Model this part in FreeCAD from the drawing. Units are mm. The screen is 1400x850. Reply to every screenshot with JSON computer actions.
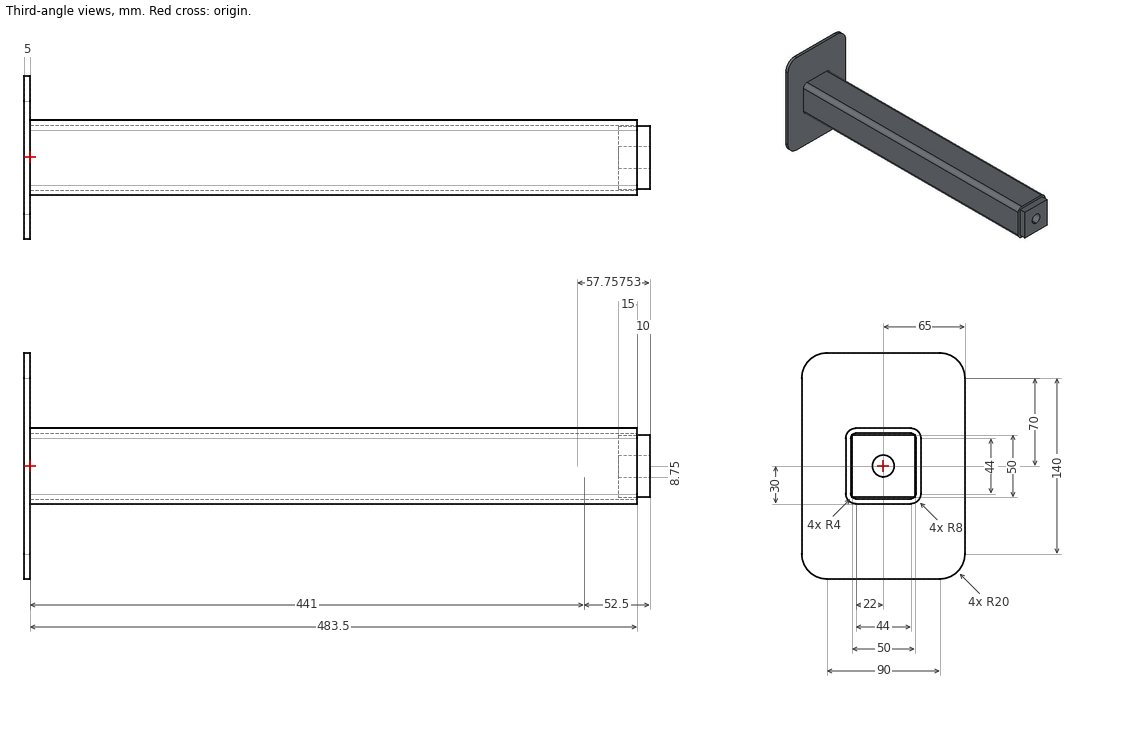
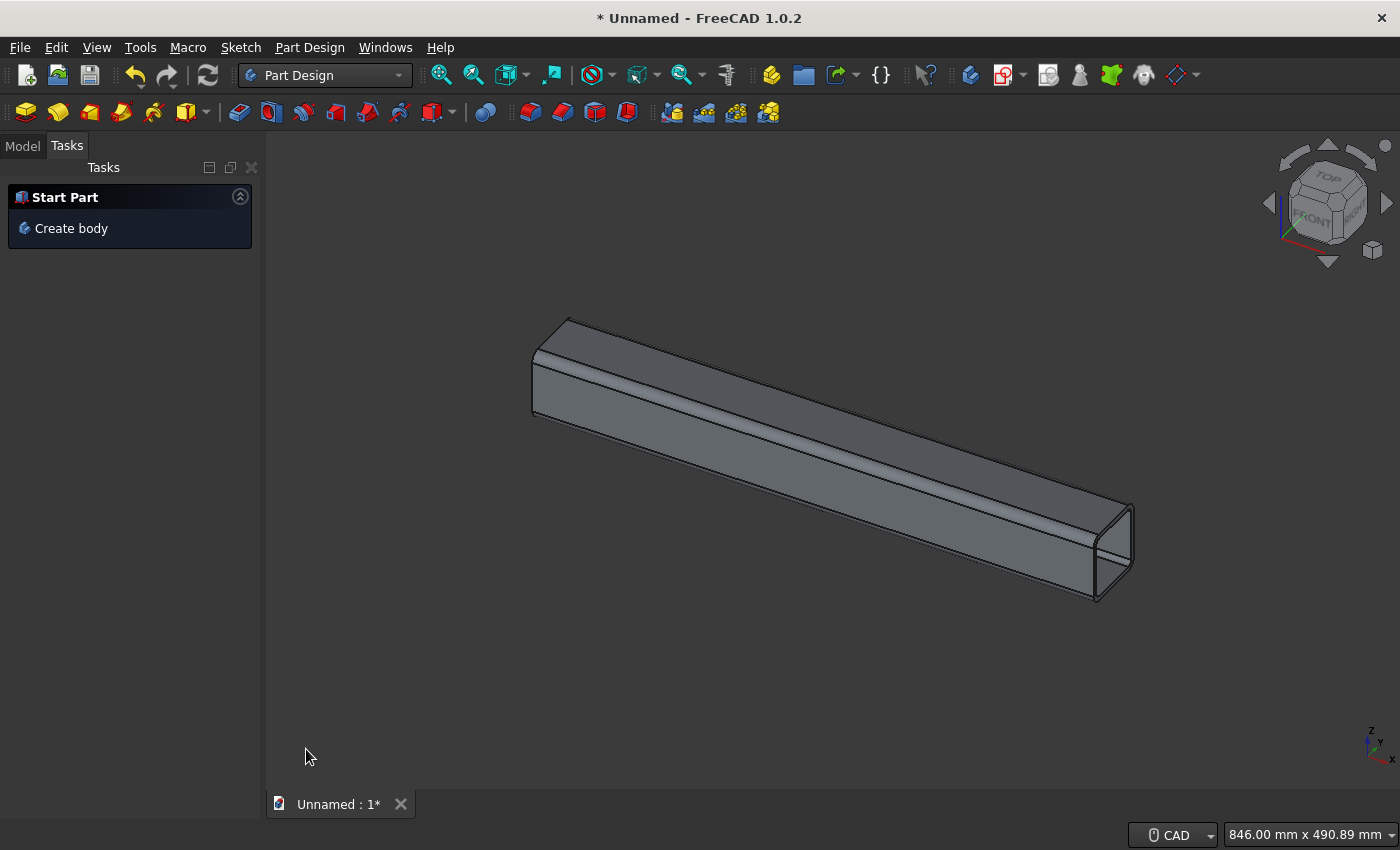
{"action": "left_click", "coordinate": [1004, 76]}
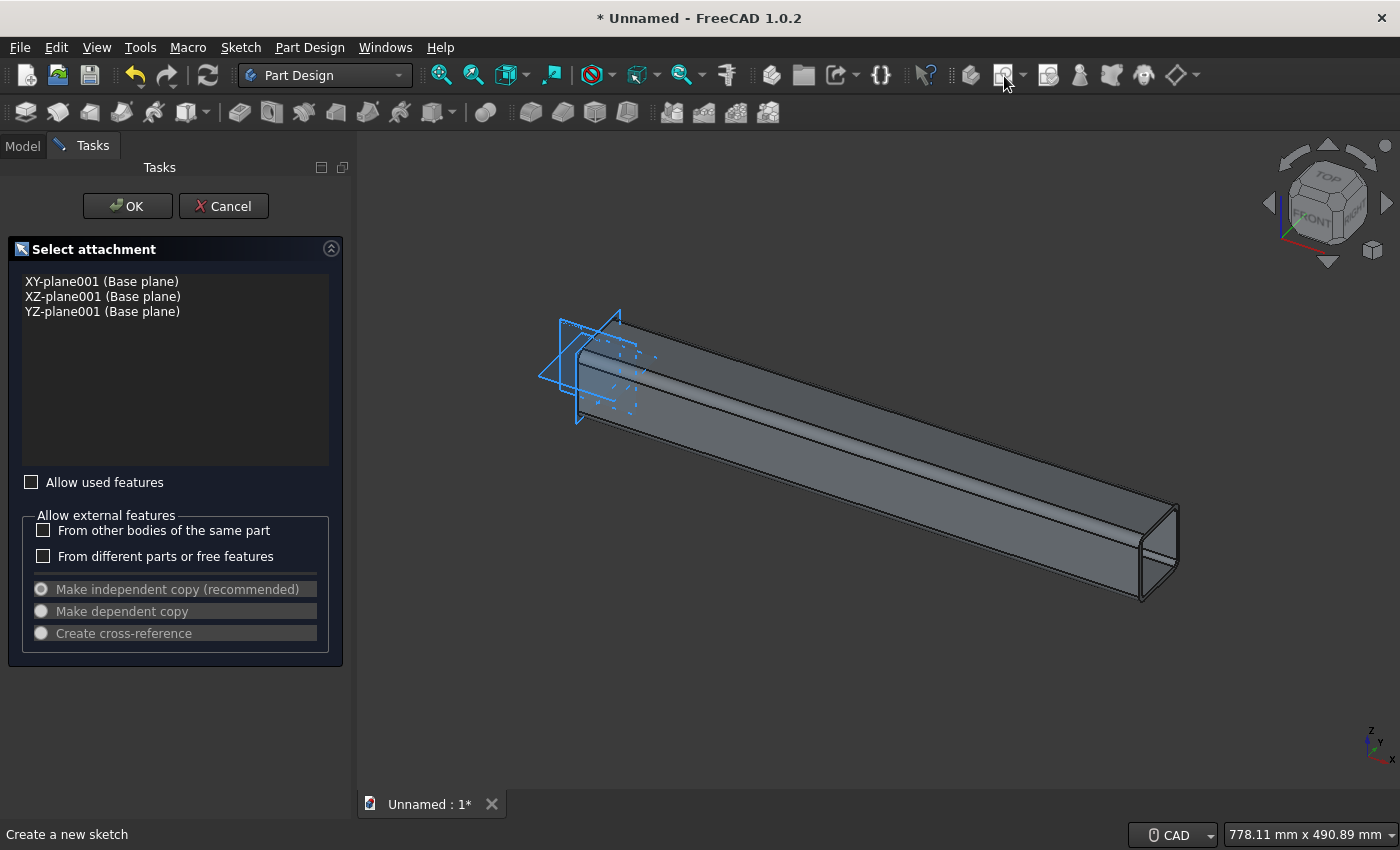
{"action": "left_click", "coordinate": [82, 312]}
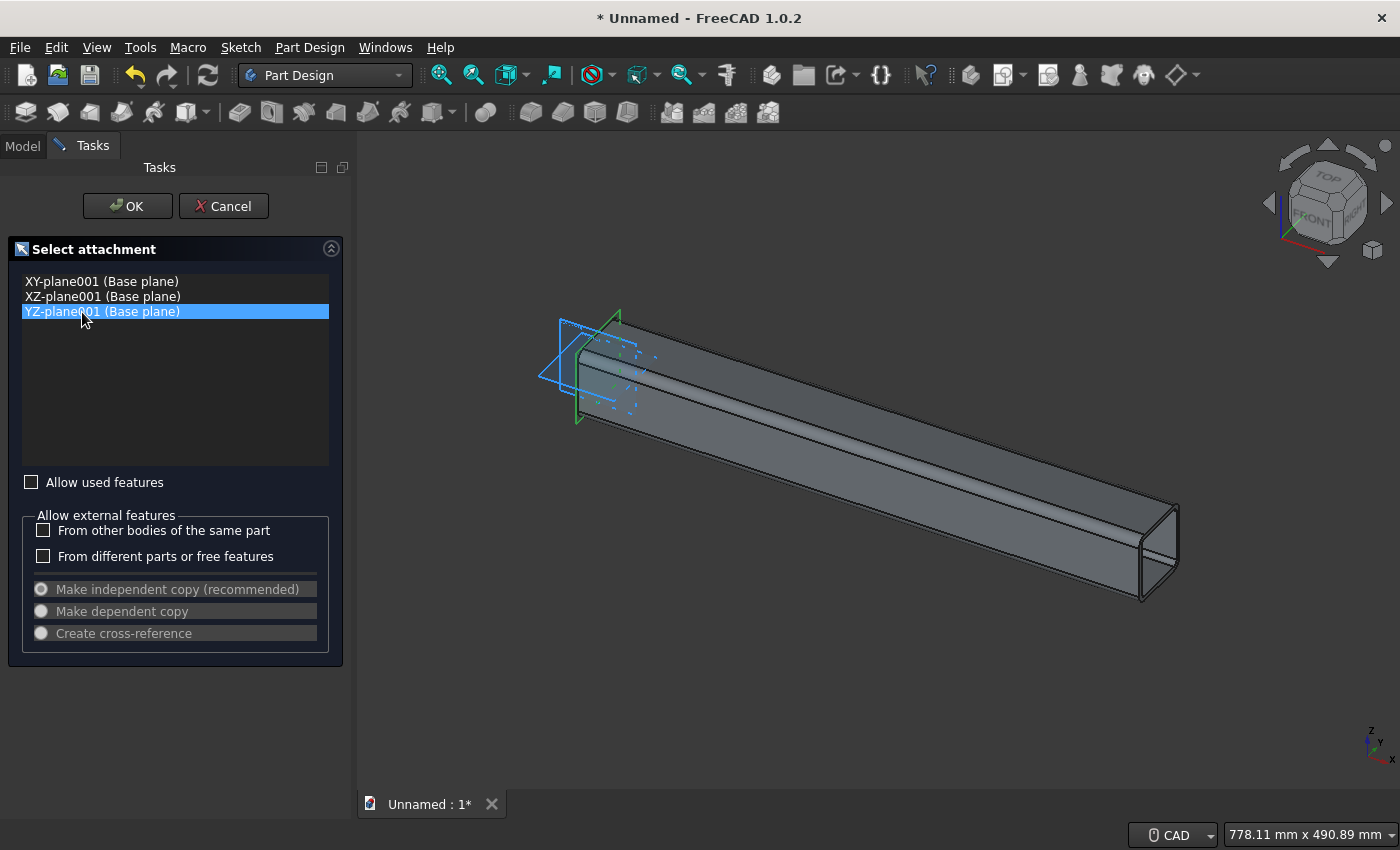
{"action": "left_click", "coordinate": [128, 206]}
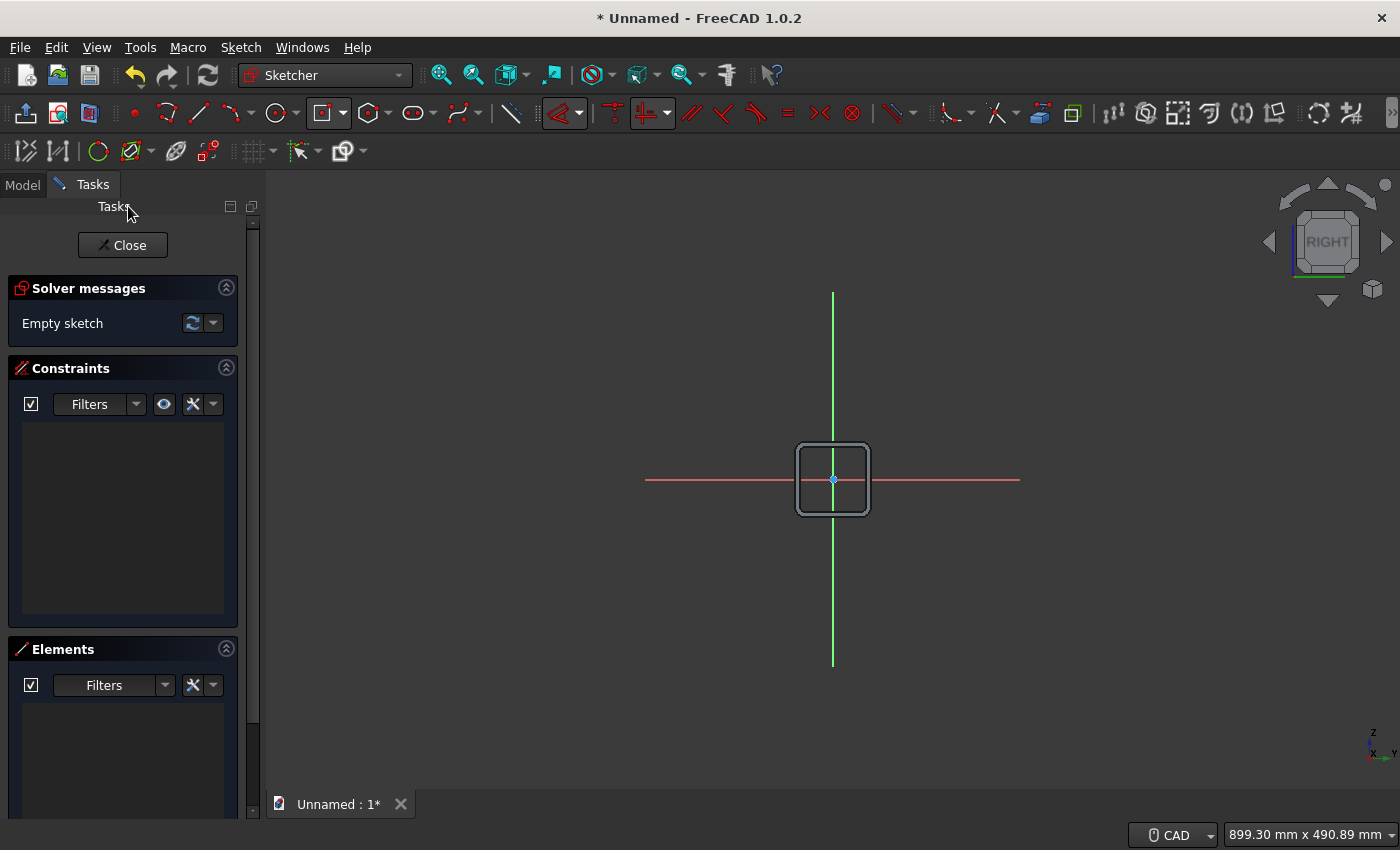
{"action": "scroll", "coordinate": [916, 480], "scroll_direction": "up", "scroll_amount": 3}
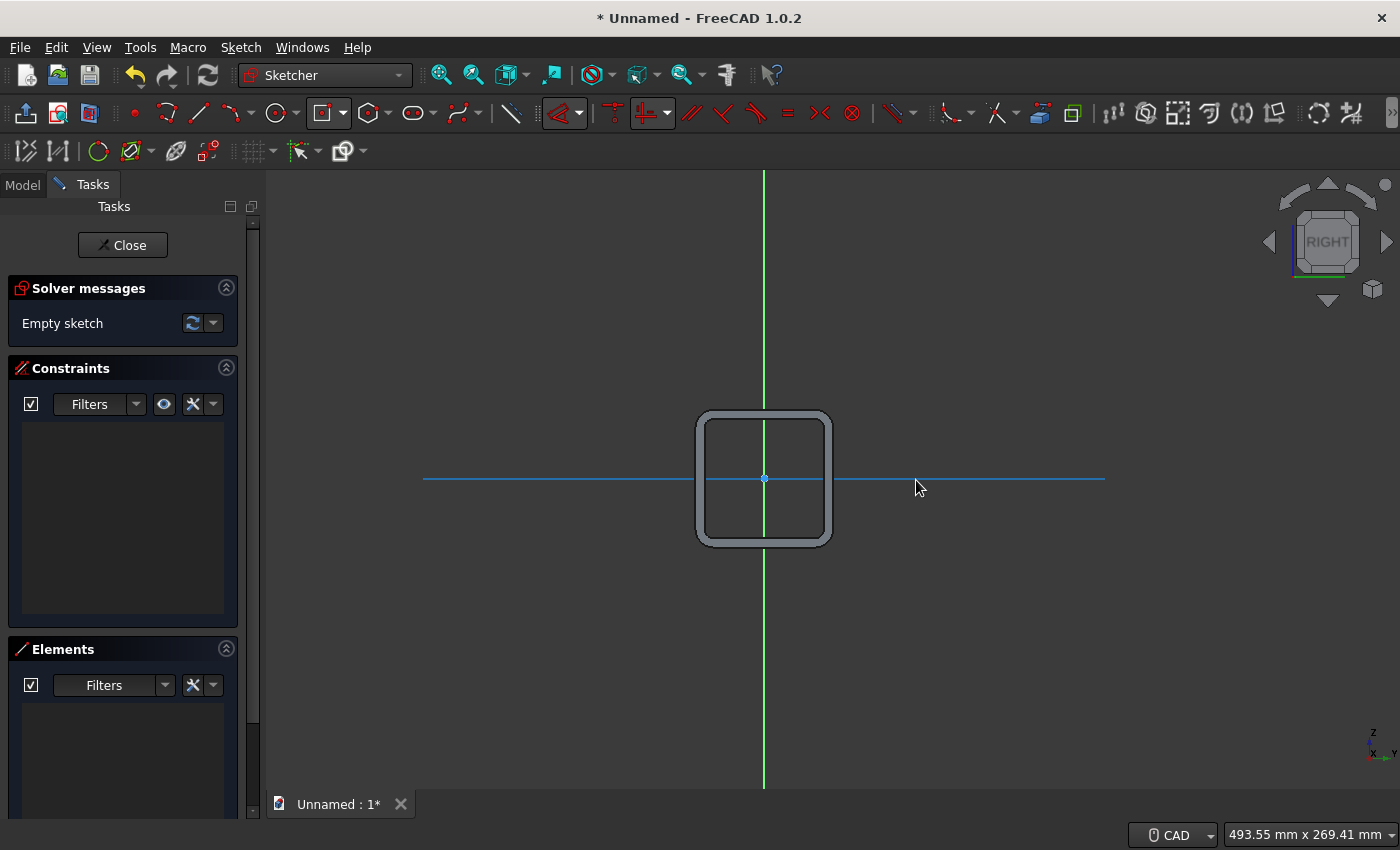
{"action": "left_click", "coordinate": [200, 114]}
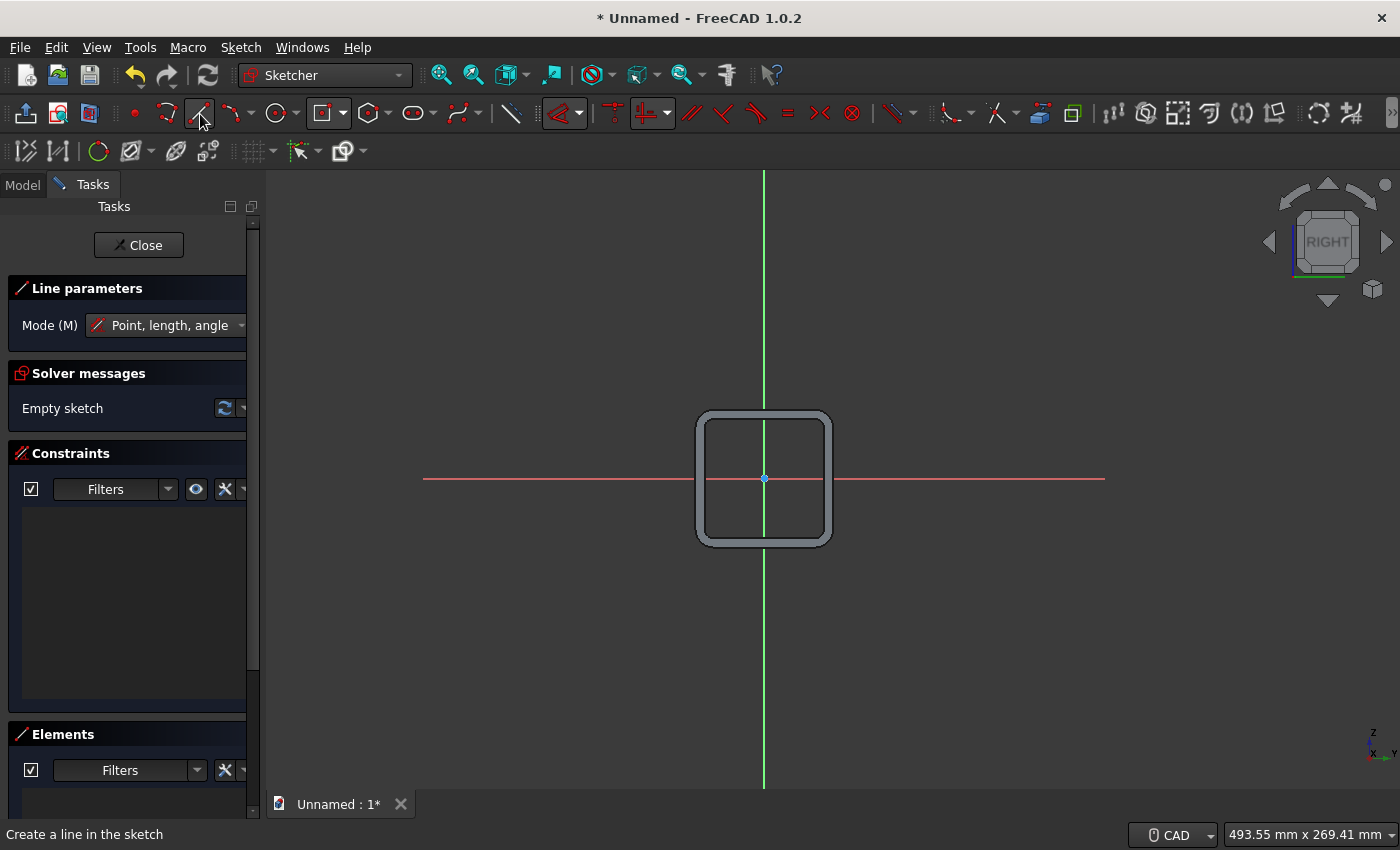
{"action": "left_click", "coordinate": [914, 318]}
{"action": "left_click", "coordinate": [914, 640]}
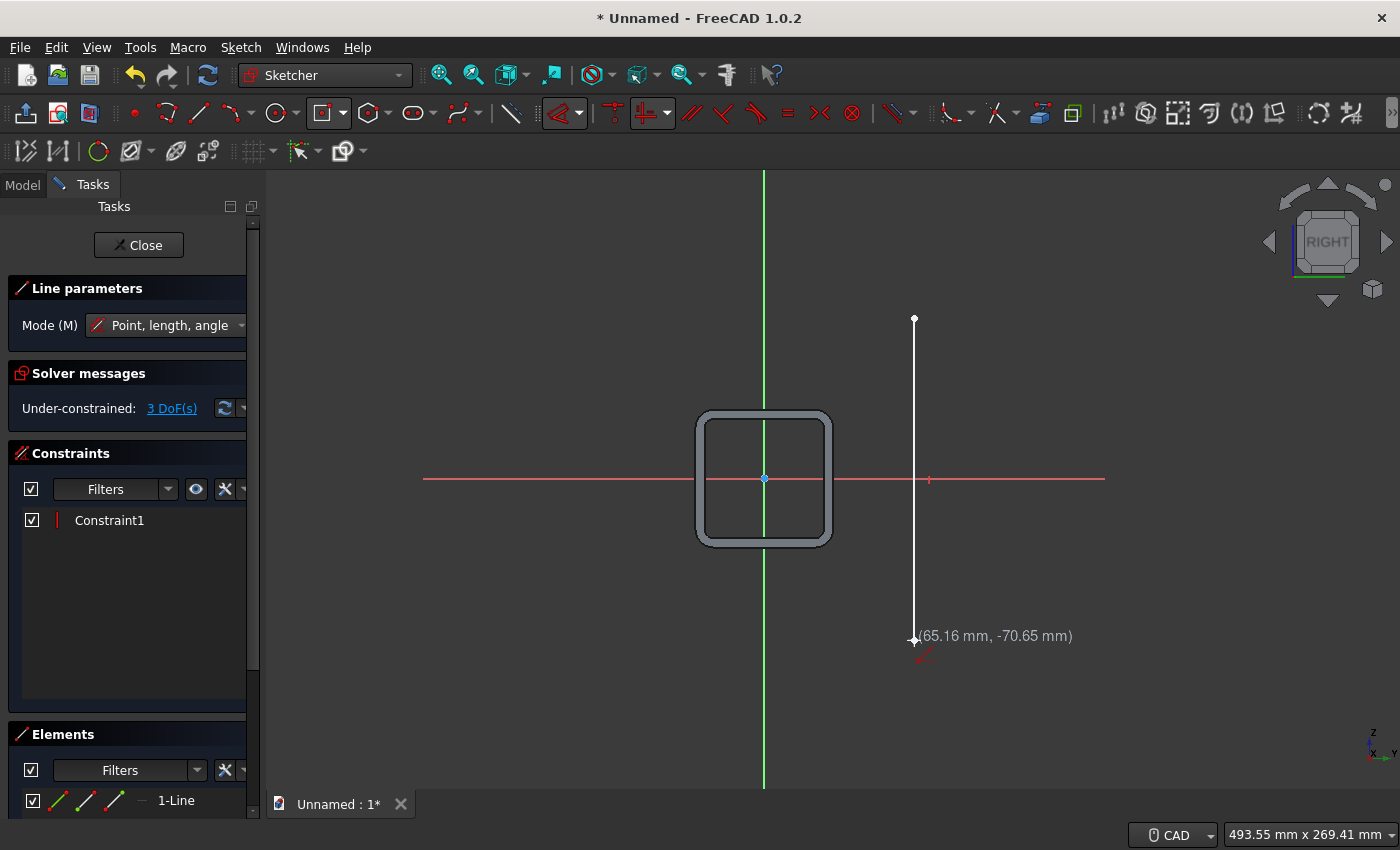
{"action": "left_click", "coordinate": [868, 685]}
{"action": "left_click", "coordinate": [661, 685]}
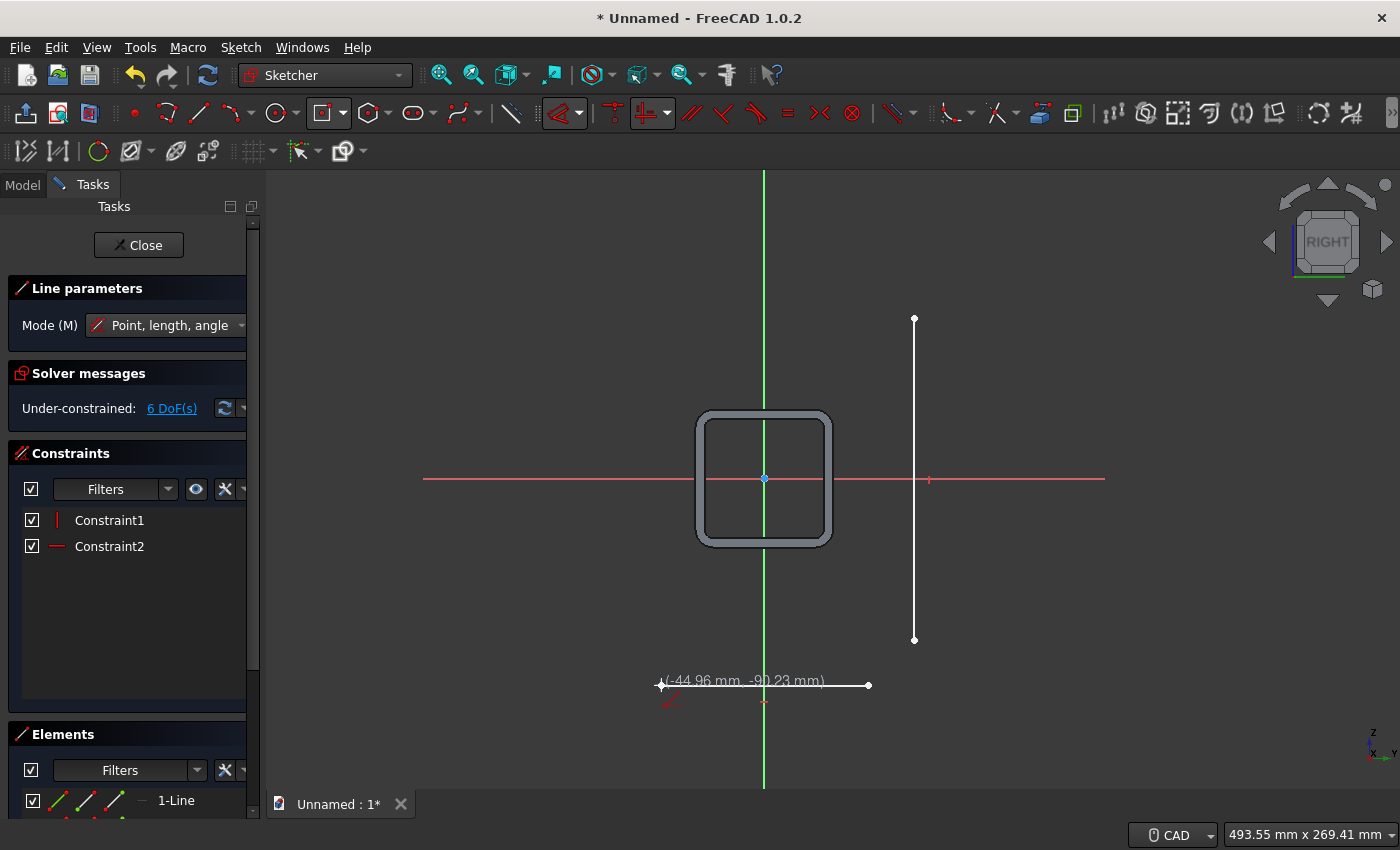
{"action": "left_click", "coordinate": [615, 640]}
{"action": "left_click", "coordinate": [615, 318]}